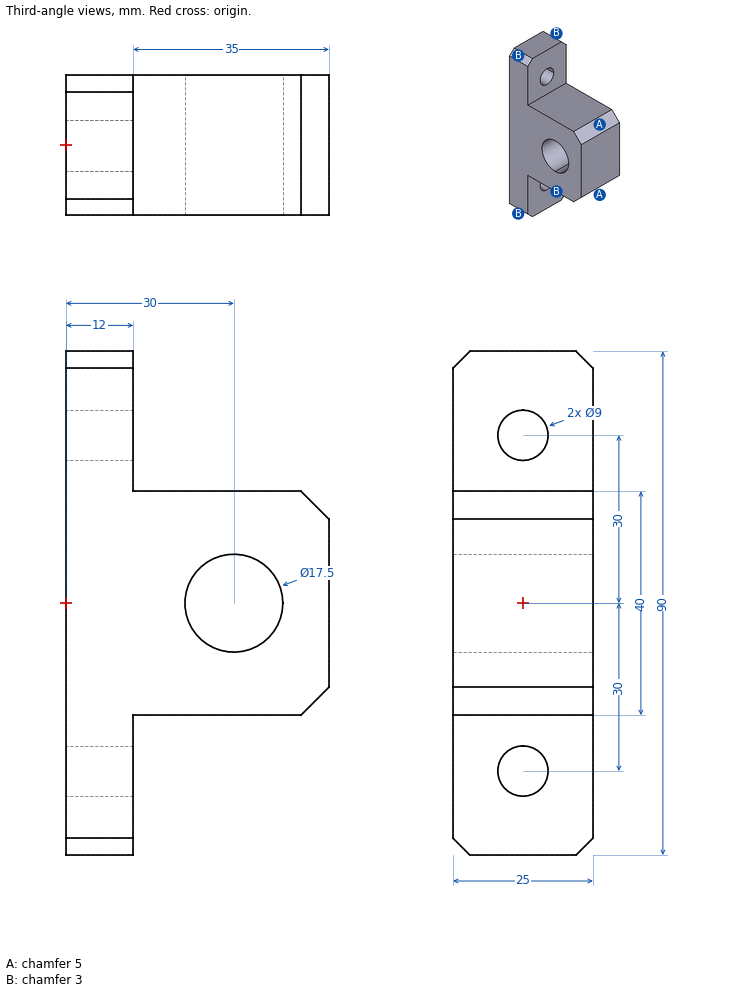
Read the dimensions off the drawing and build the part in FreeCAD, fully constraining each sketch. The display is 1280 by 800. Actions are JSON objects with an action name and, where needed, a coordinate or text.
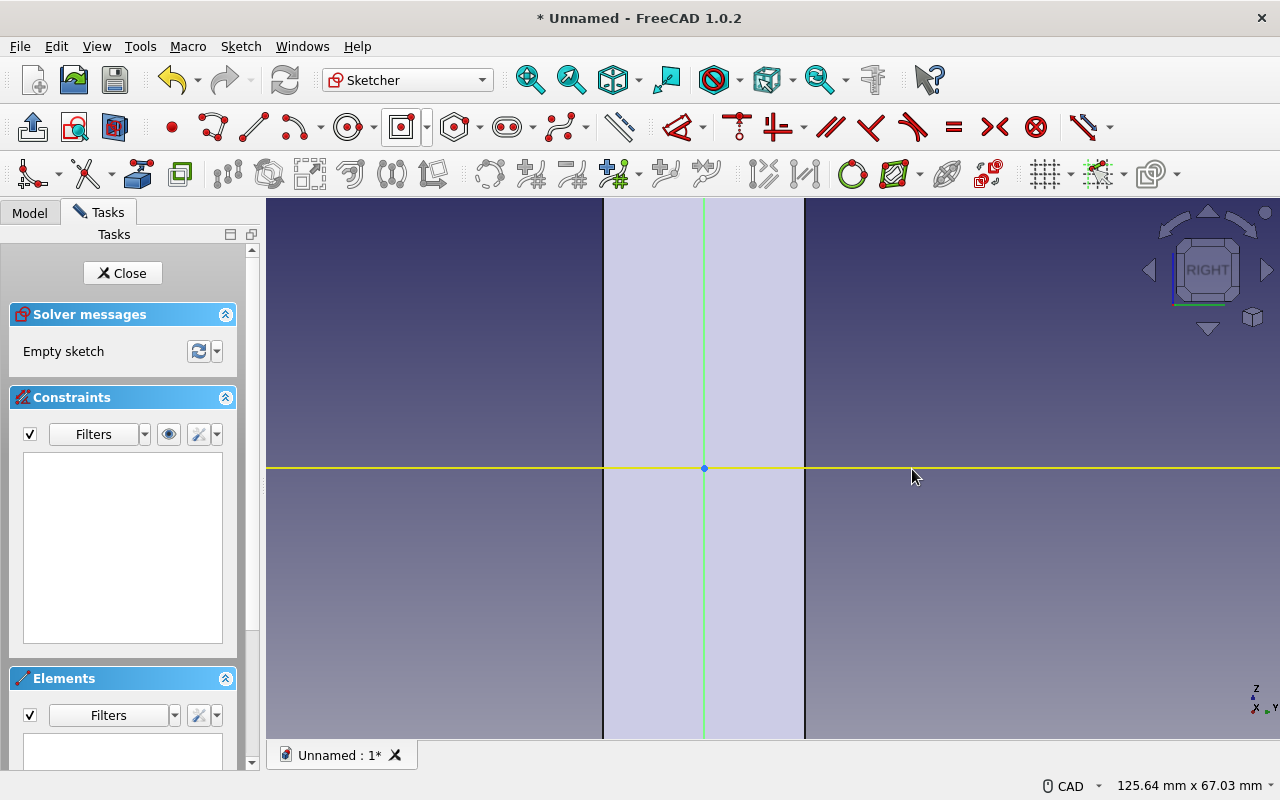
{"action": "left_click", "coordinate": [400, 128]}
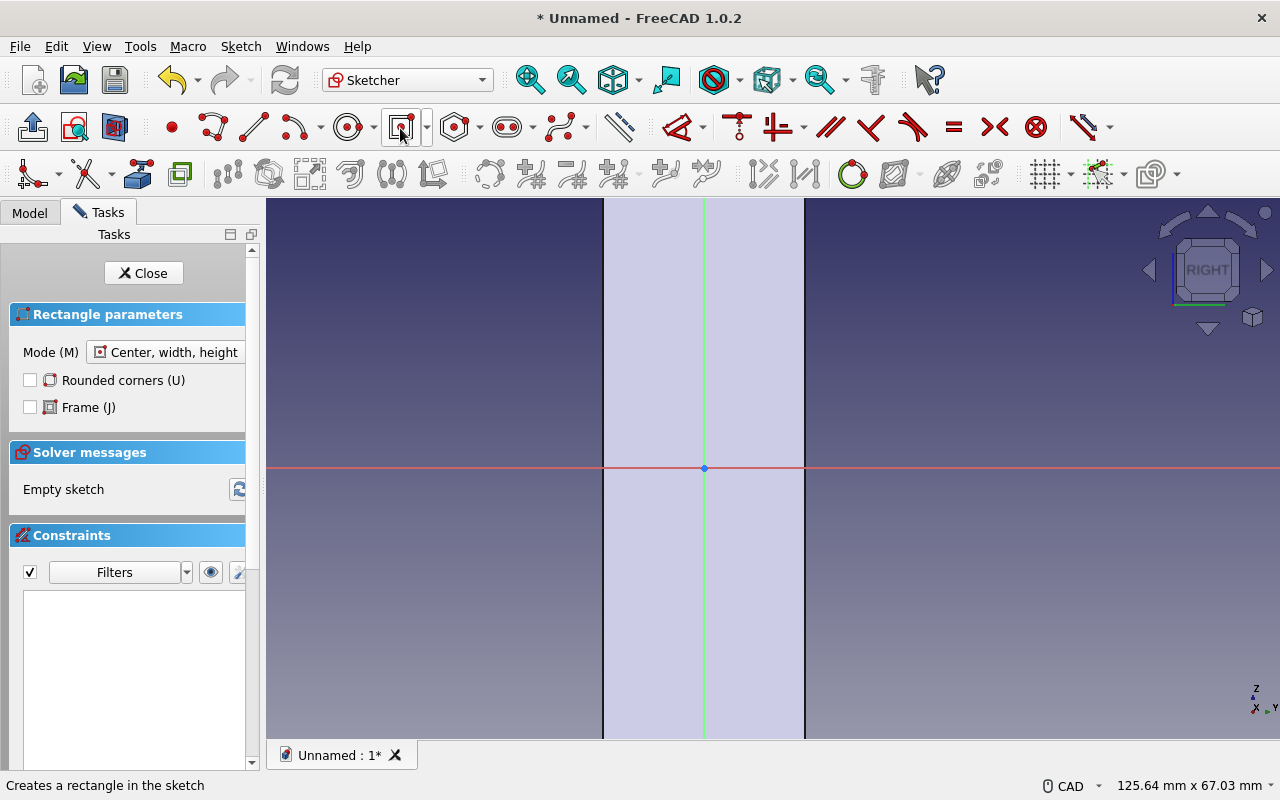
{"action": "left_click", "coordinate": [704, 468]}
{"action": "left_click", "coordinate": [805, 307]}
{"action": "key", "text": "Escape"}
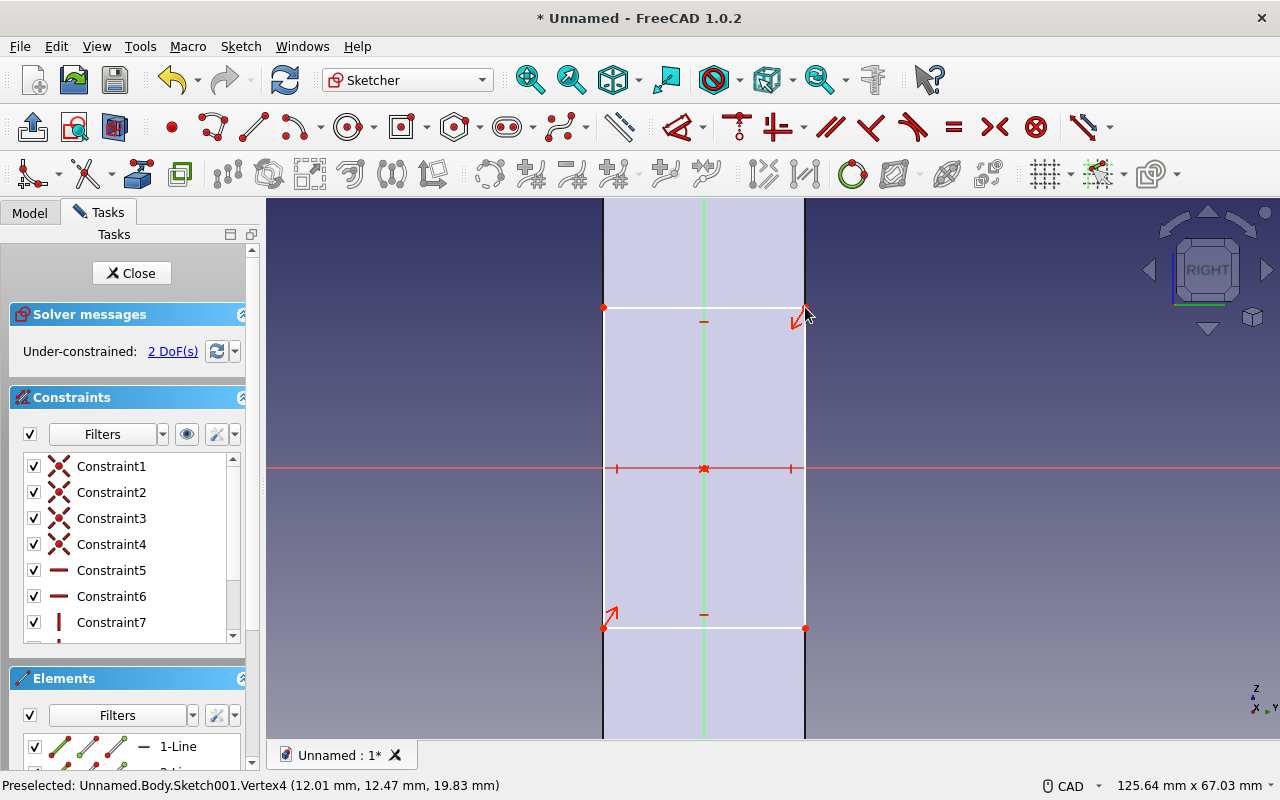
{"action": "key", "text": "d"}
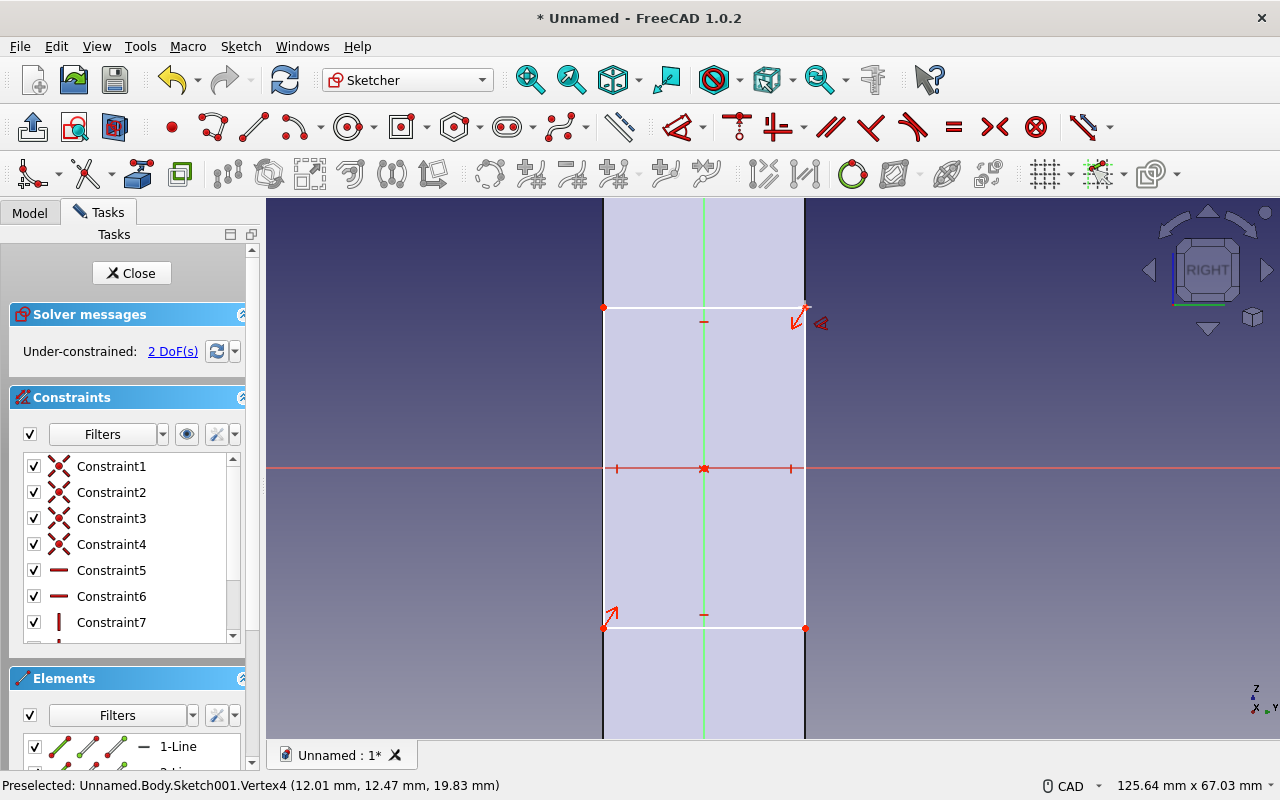
{"action": "left_click", "coordinate": [664, 628]}
{"action": "left_click", "coordinate": [658, 662]}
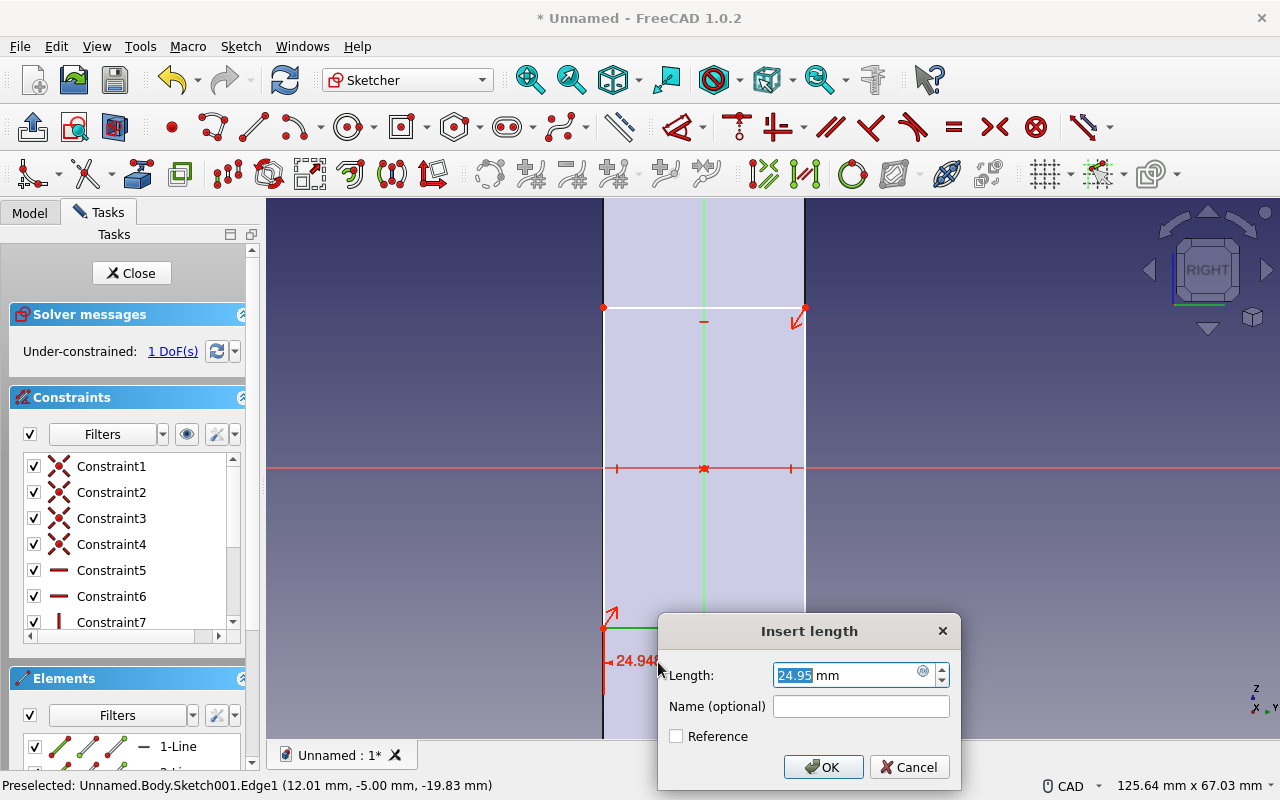
{"action": "type", "text": "25"}
{"action": "key", "text": "Return"}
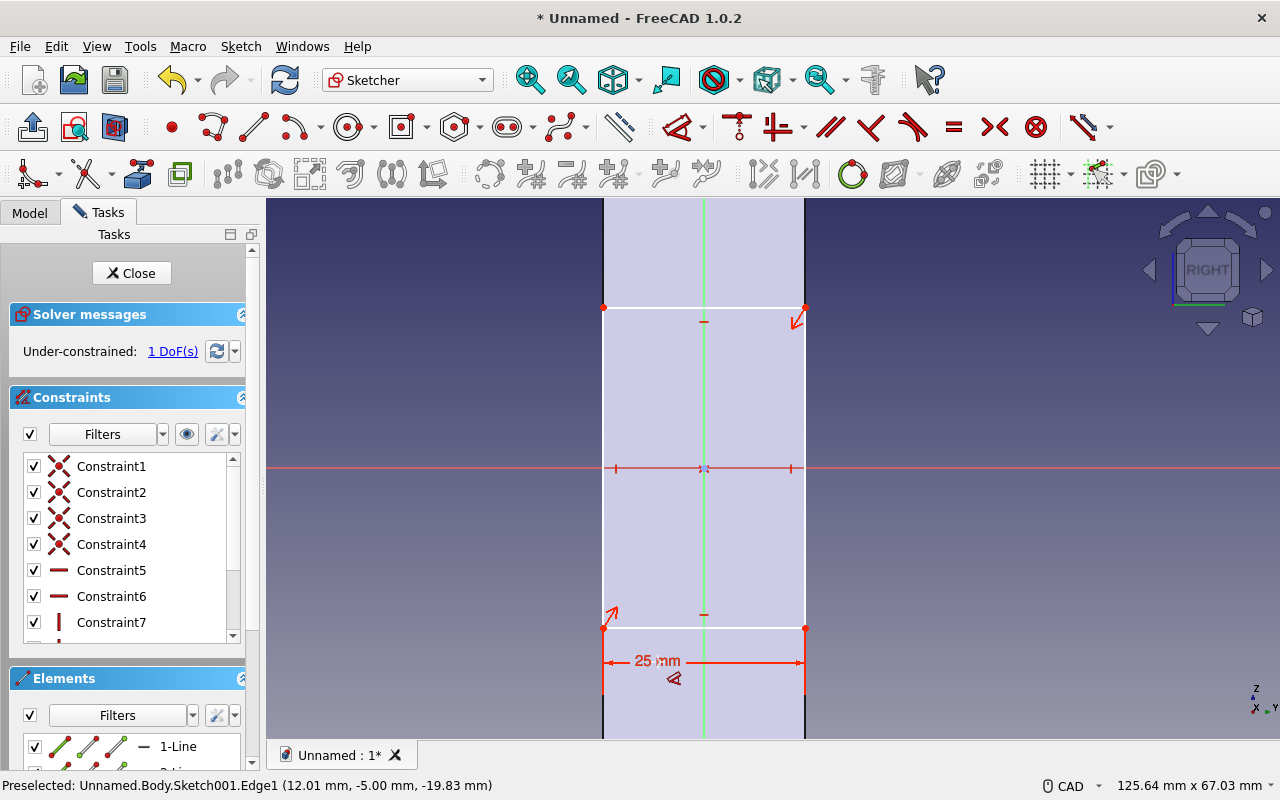
{"action": "left_click", "coordinate": [805, 532]}
{"action": "left_click", "coordinate": [839, 394]}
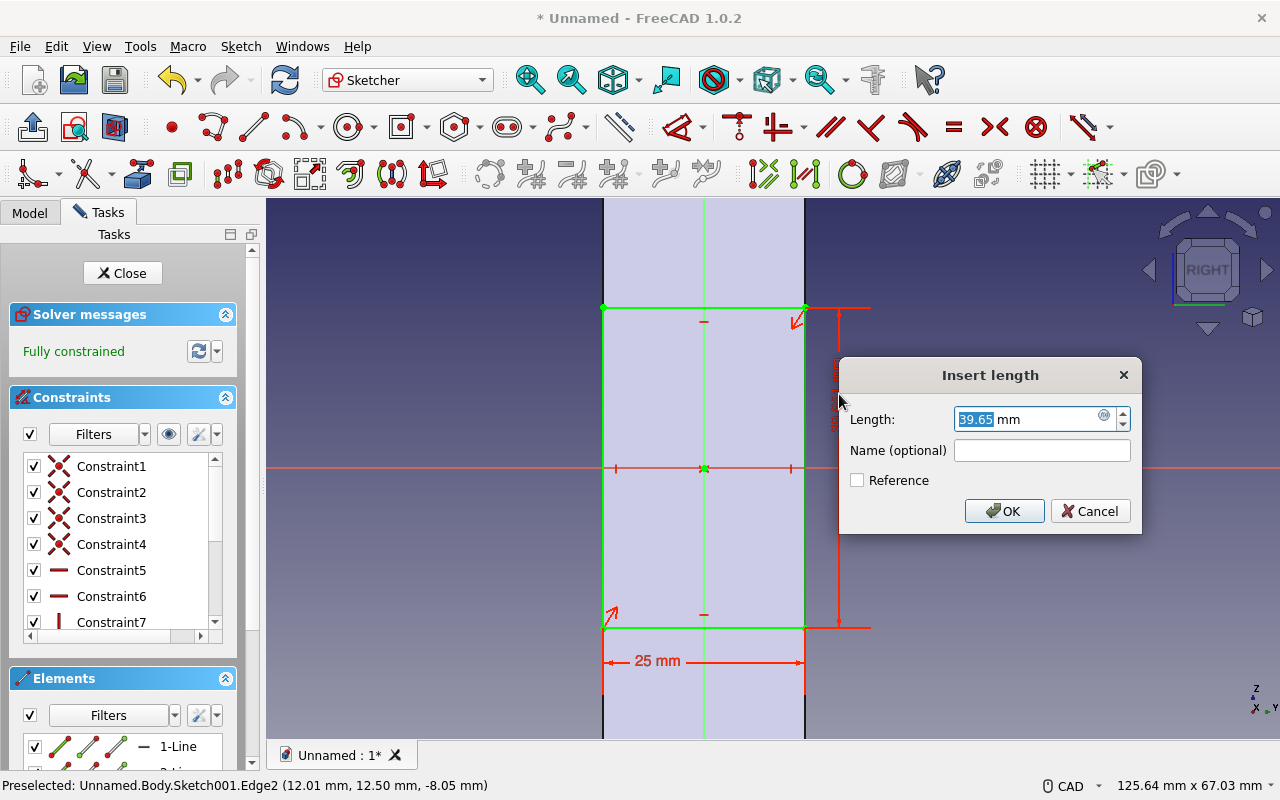
{"action": "type", "text": "40"}
{"action": "key", "text": "Return"}
{"action": "key", "text": "Escape"}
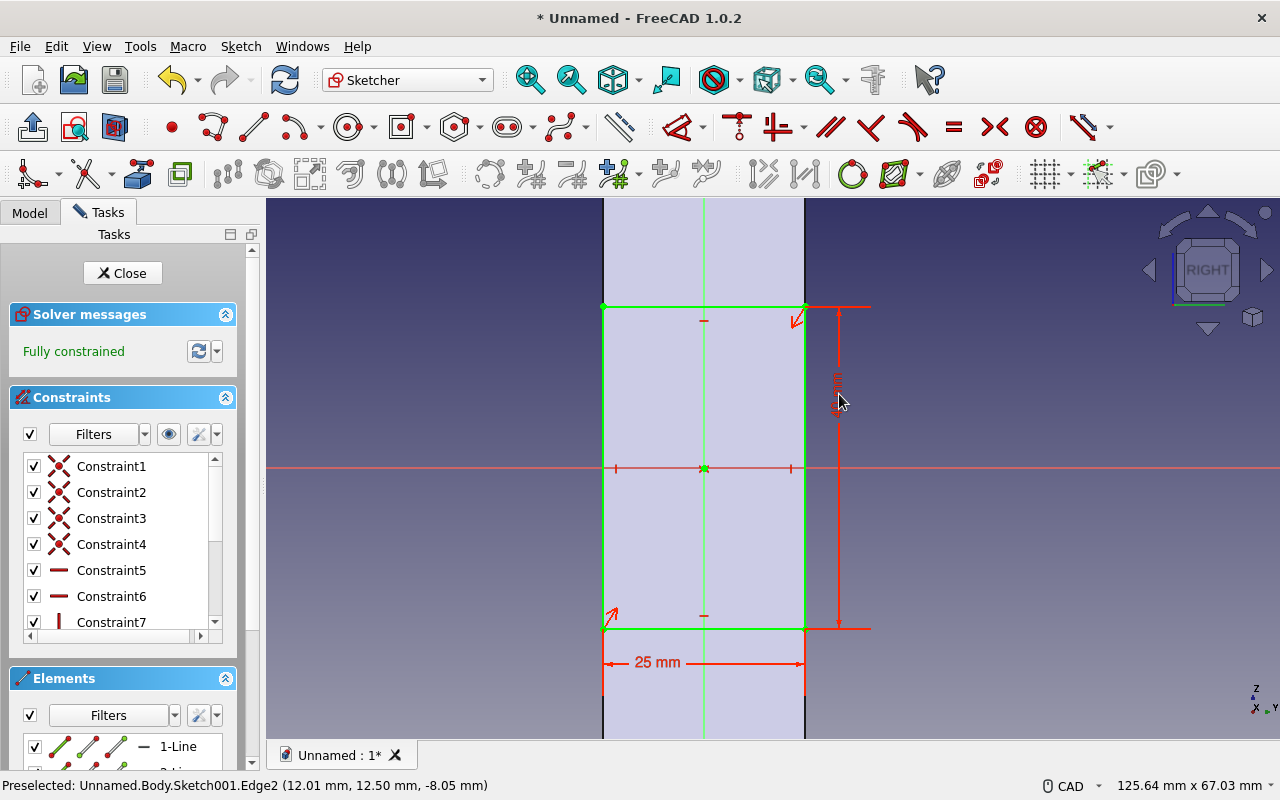
{"action": "left_click", "coordinate": [123, 273]}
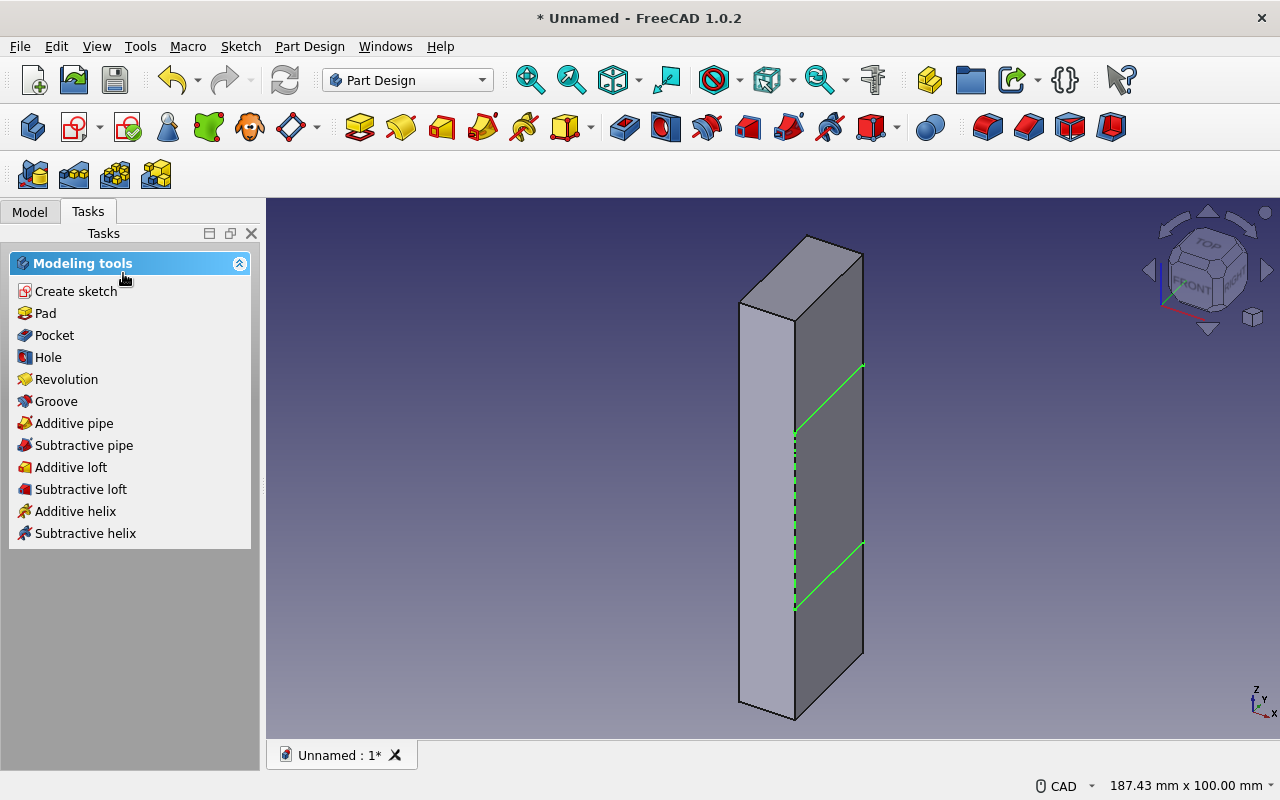
{"action": "left_click", "coordinate": [360, 128]}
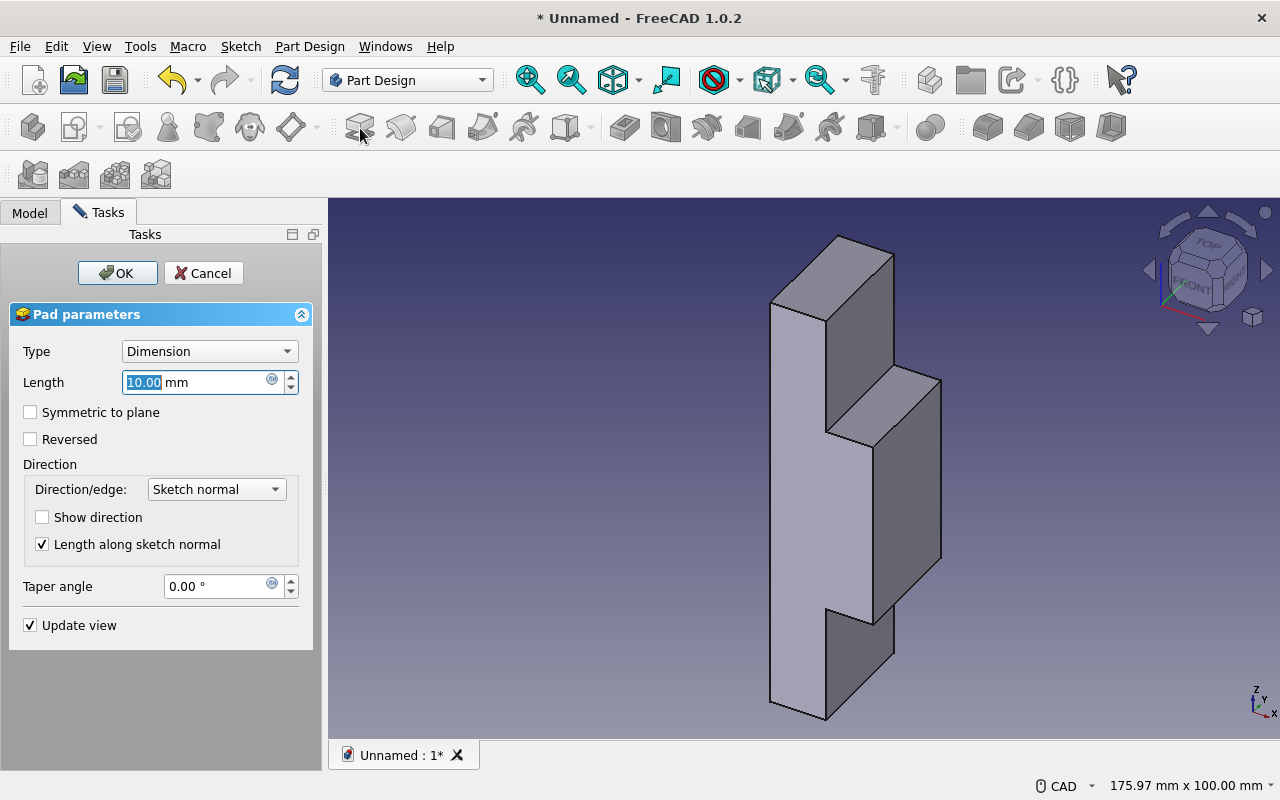
{"action": "type", "text": "35"}
{"action": "key", "text": "Tab"}